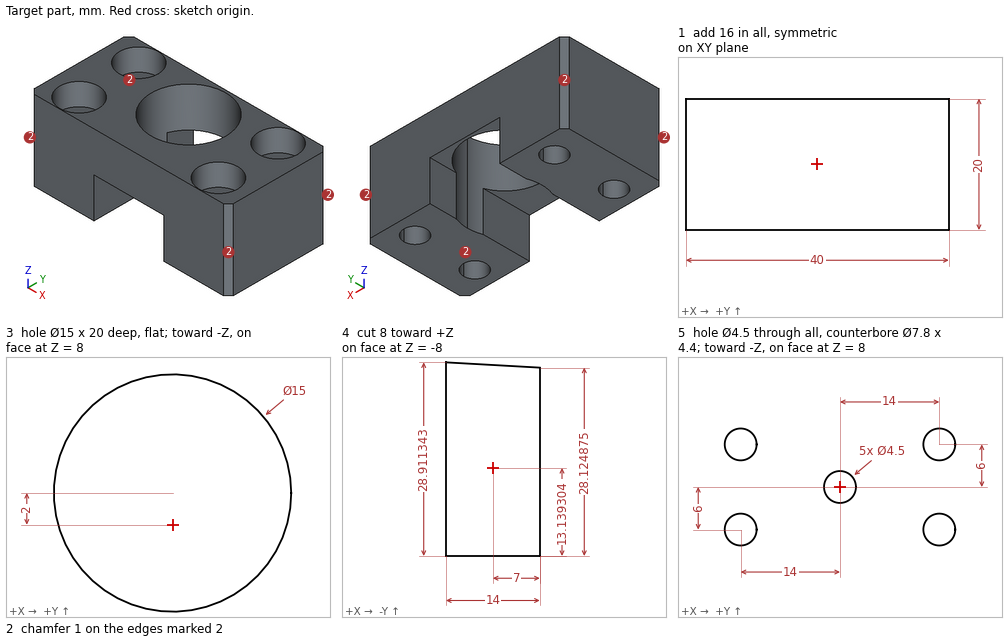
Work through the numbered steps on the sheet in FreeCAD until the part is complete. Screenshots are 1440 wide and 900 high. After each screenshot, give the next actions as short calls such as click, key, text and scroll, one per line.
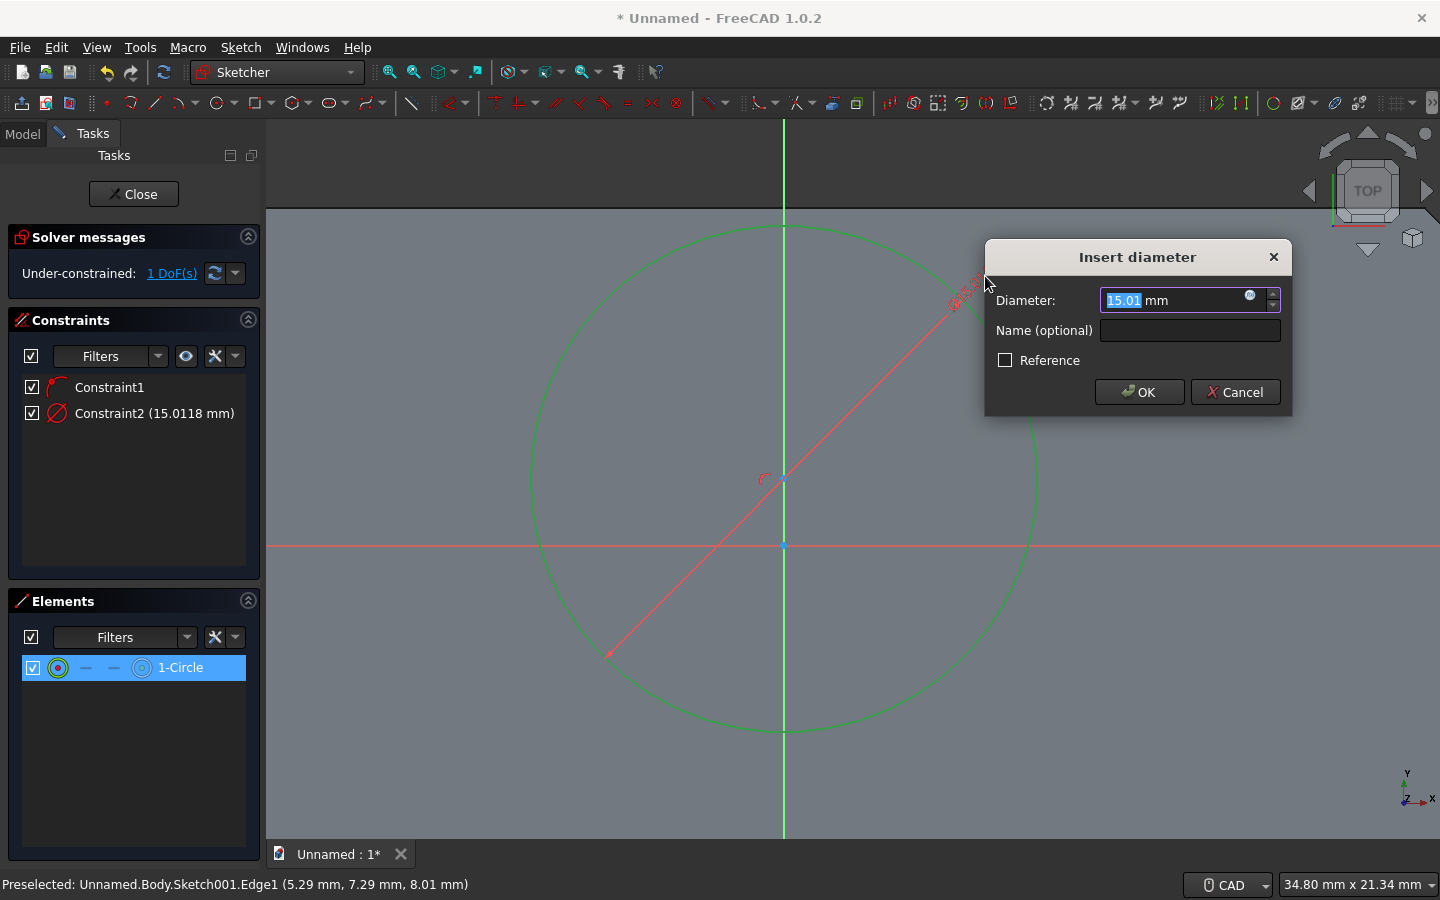
text(15)
key(Return)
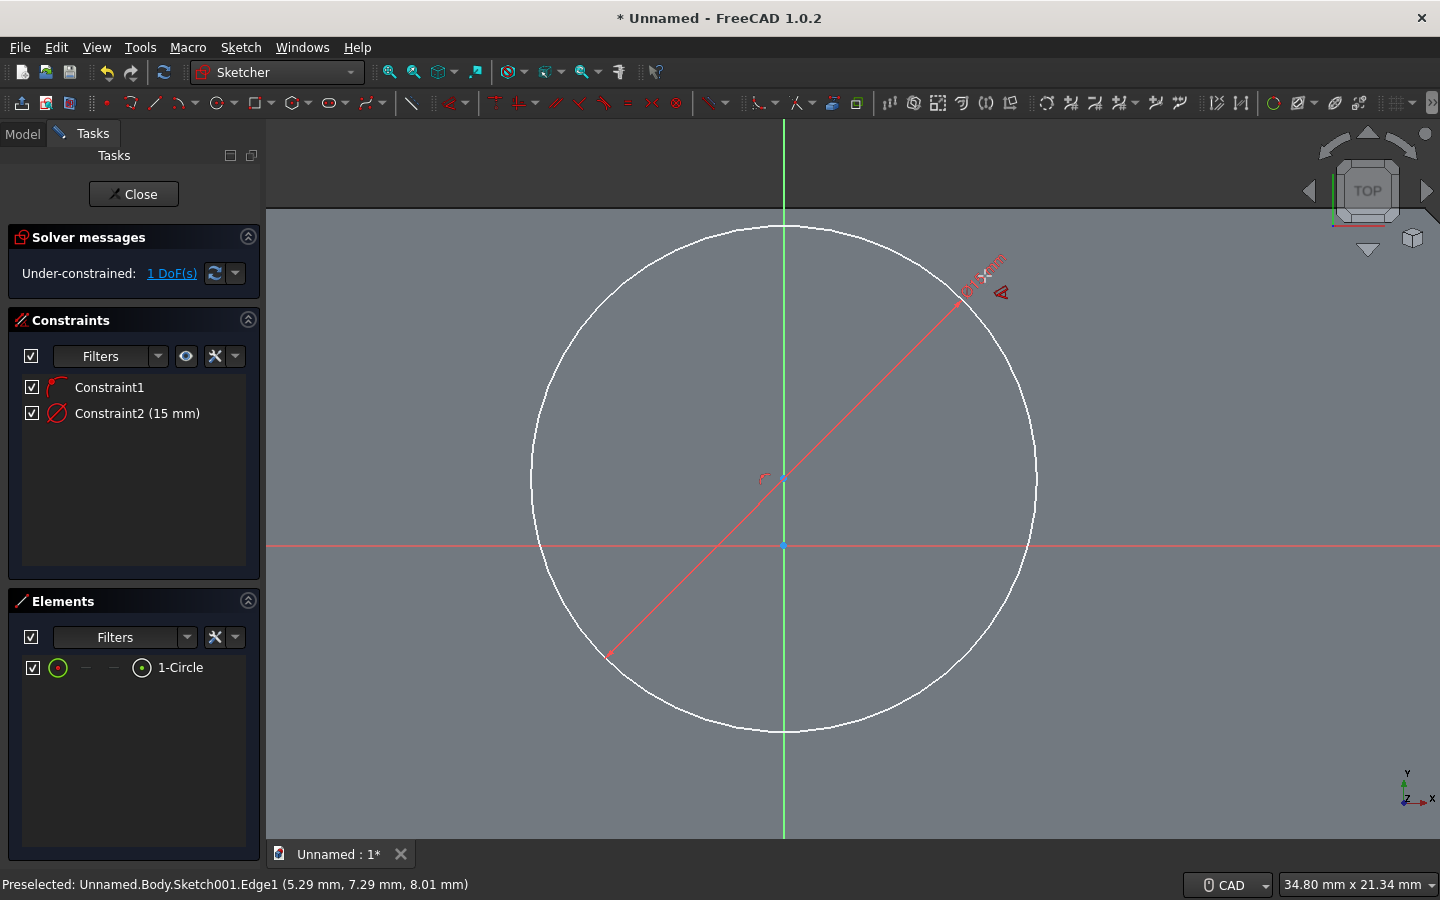
click(784, 479)
click(818, 512)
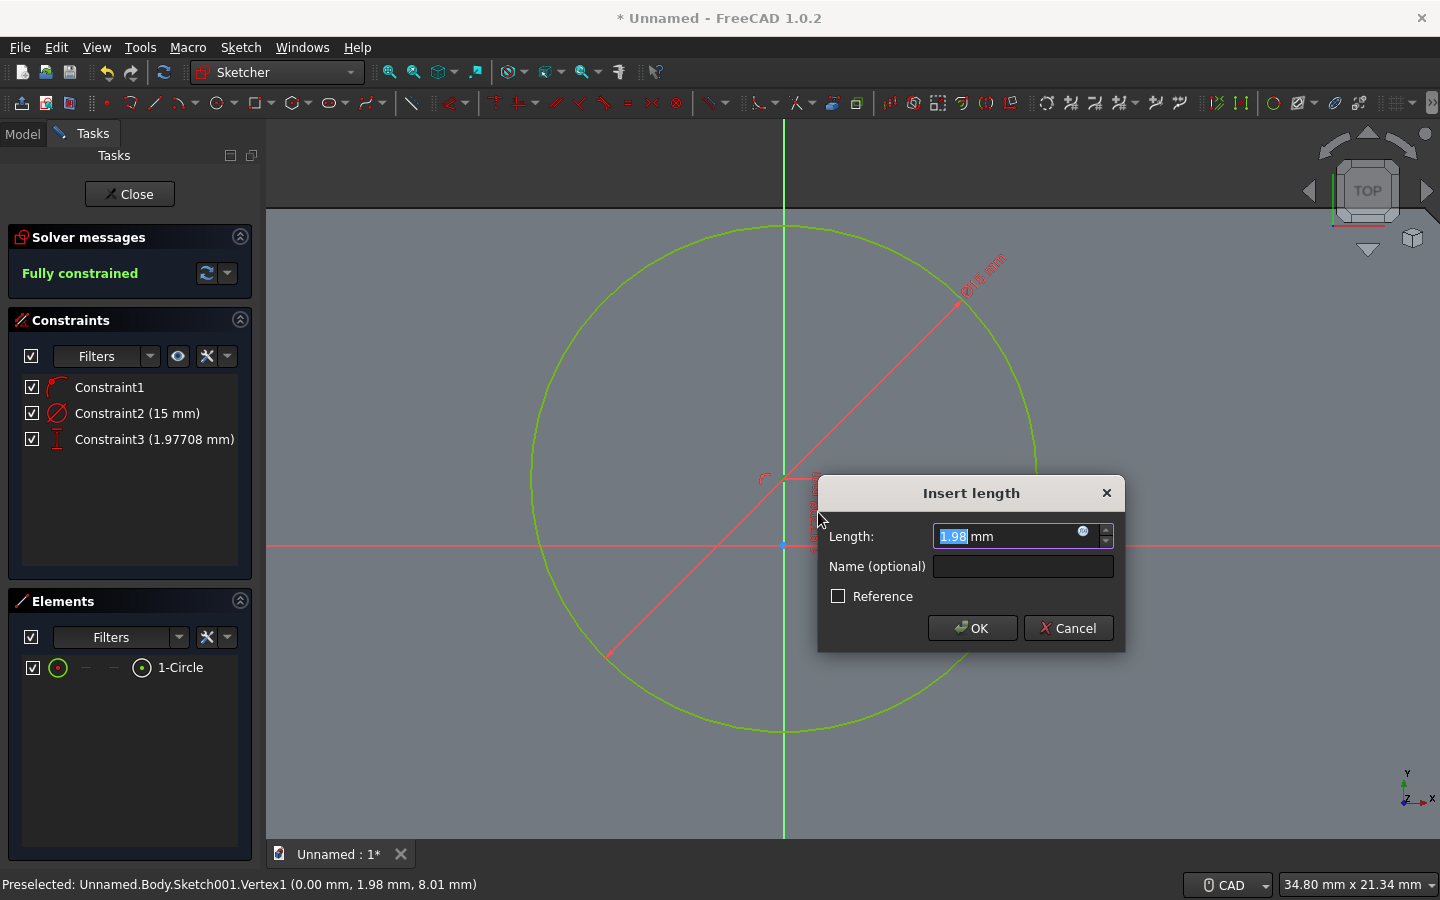
text(2)
key(Return)
key(Escape)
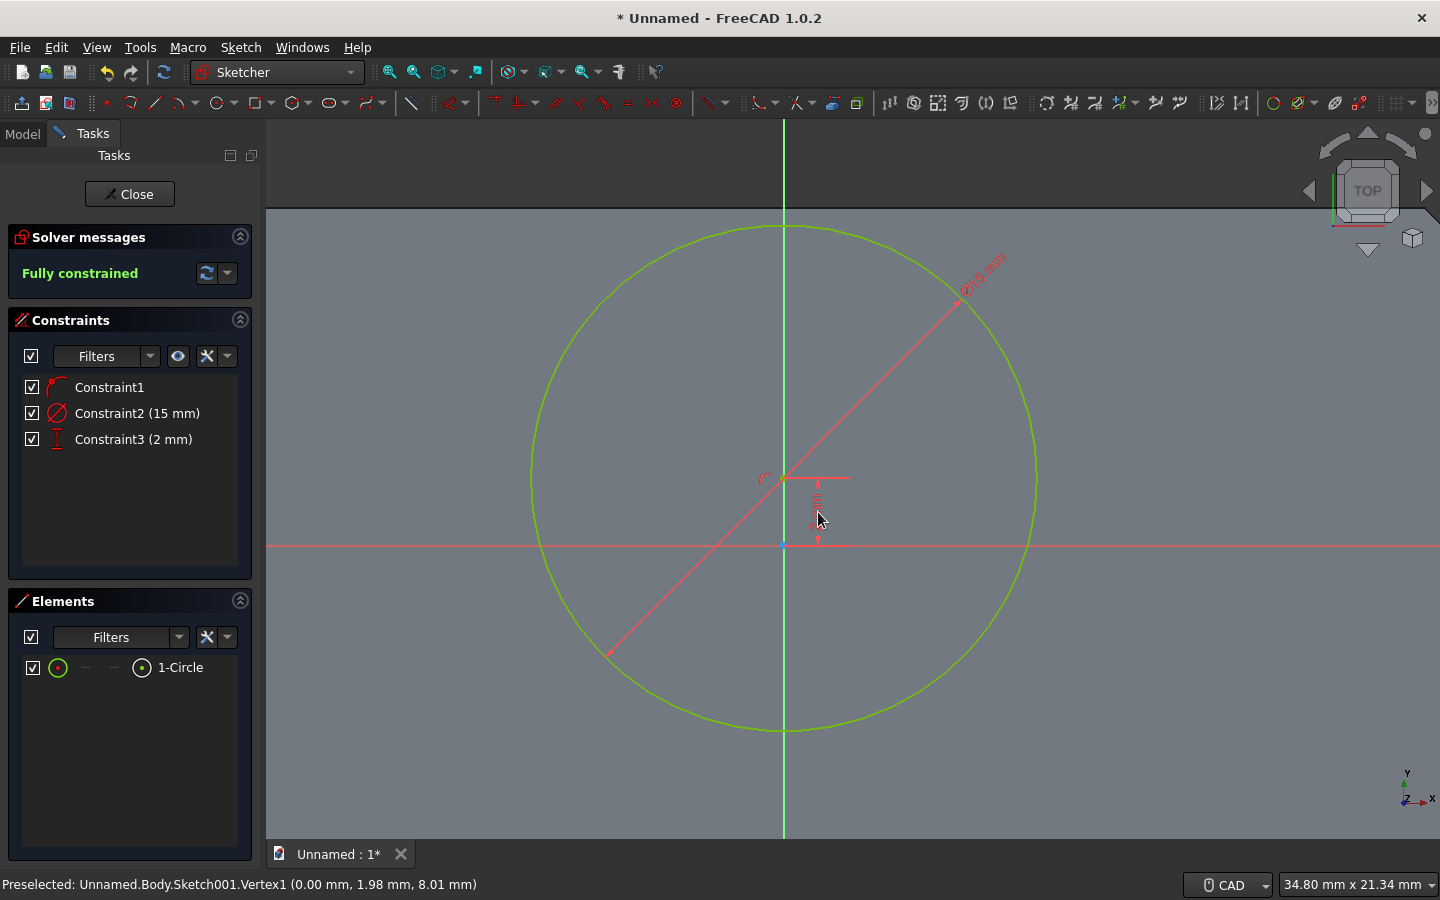
click(130, 194)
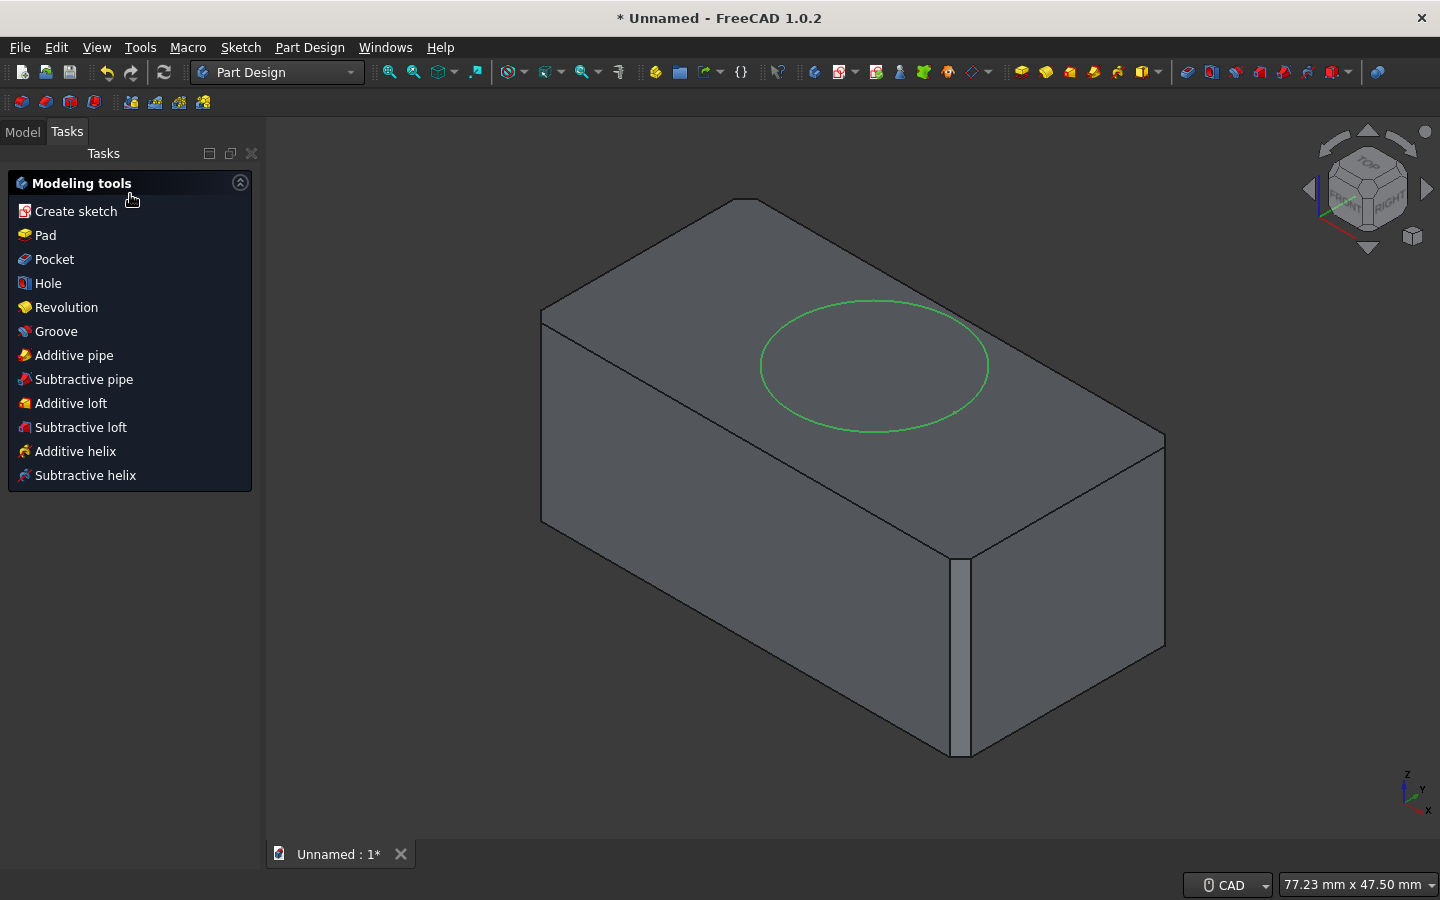
click(1212, 72)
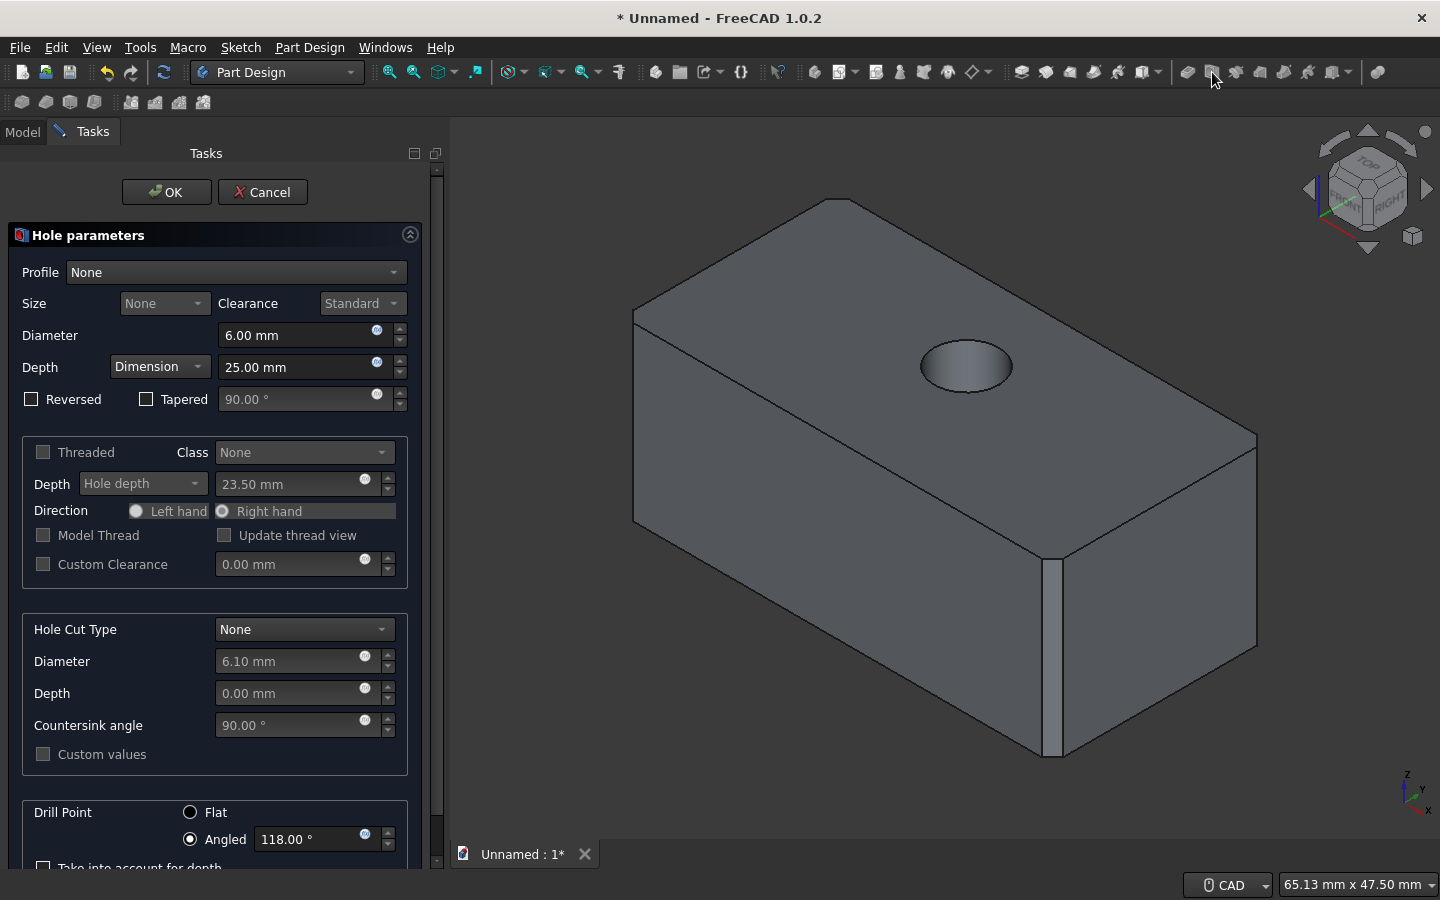
triple_click(305, 335)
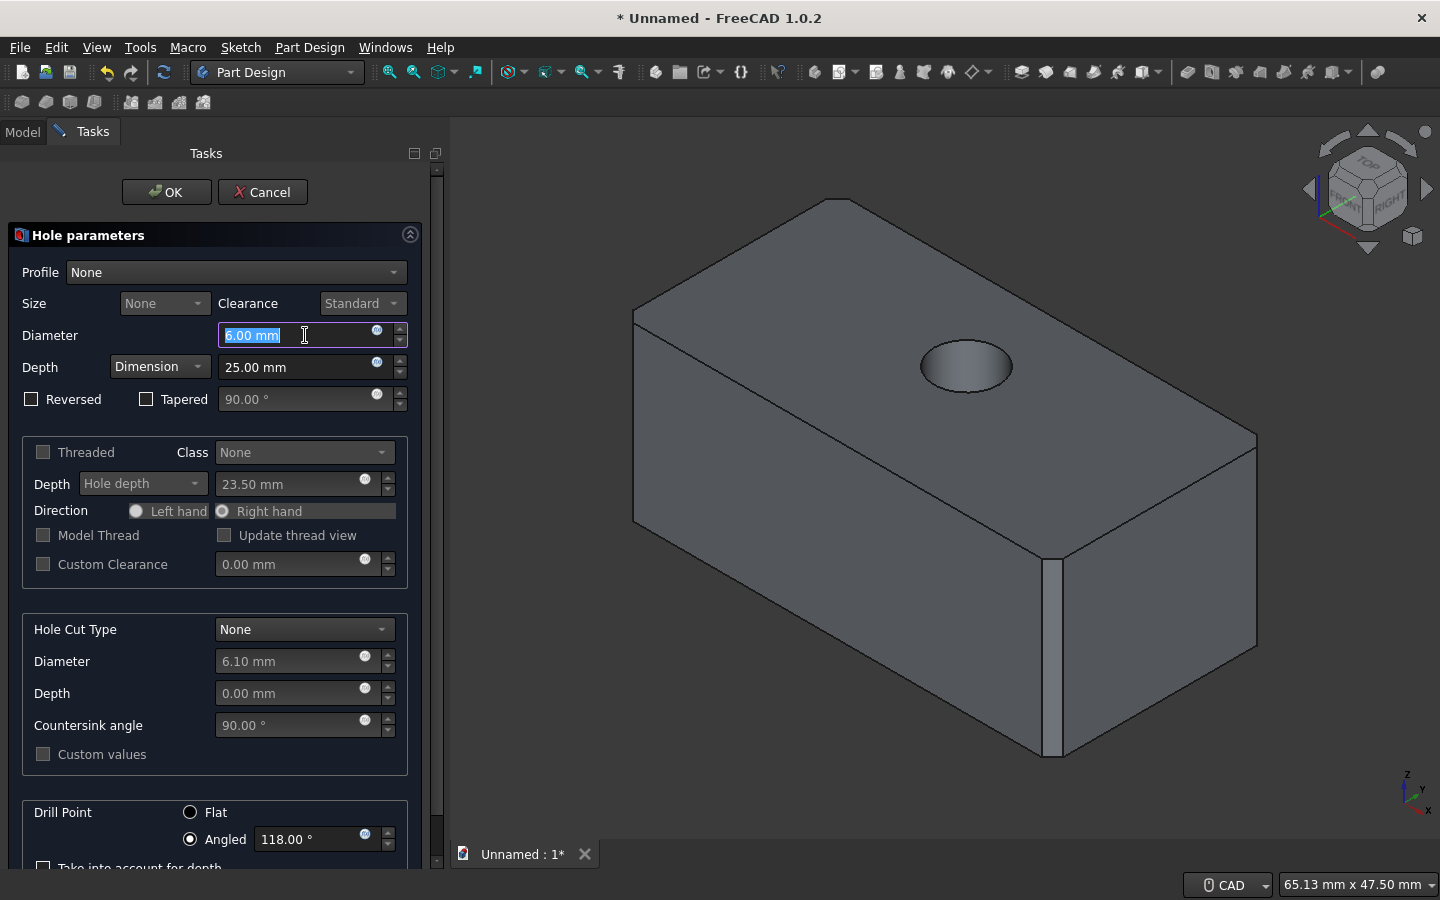
text(15)
key(Tab)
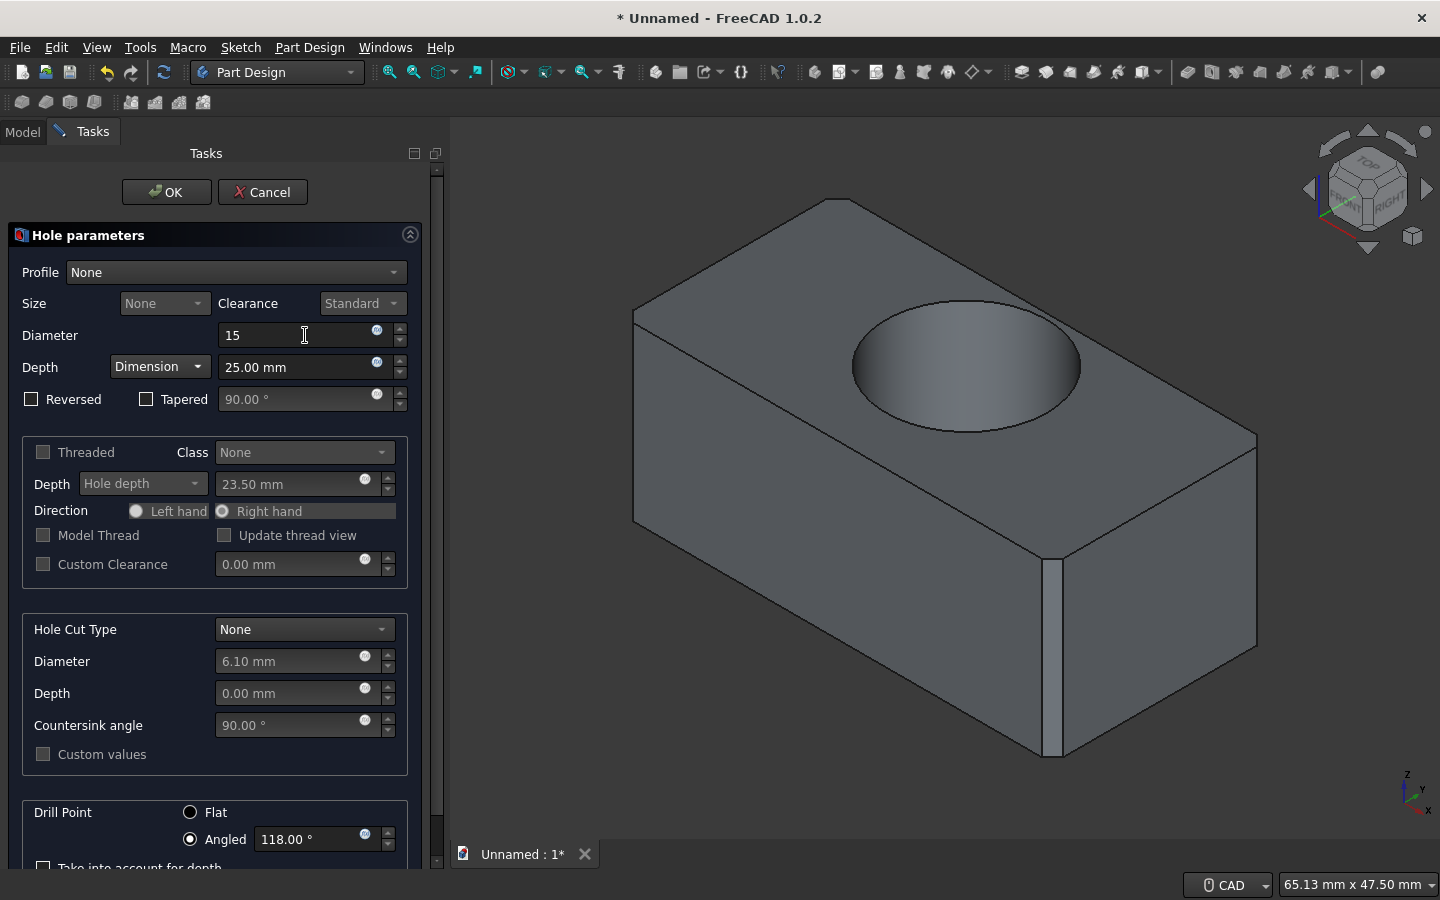
triple_click(305, 367)